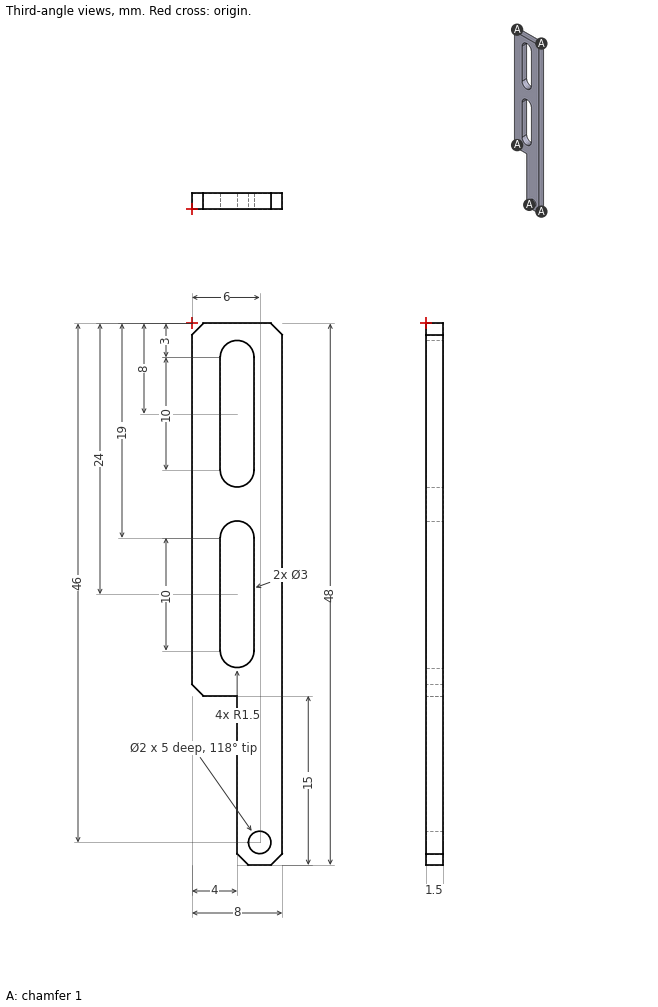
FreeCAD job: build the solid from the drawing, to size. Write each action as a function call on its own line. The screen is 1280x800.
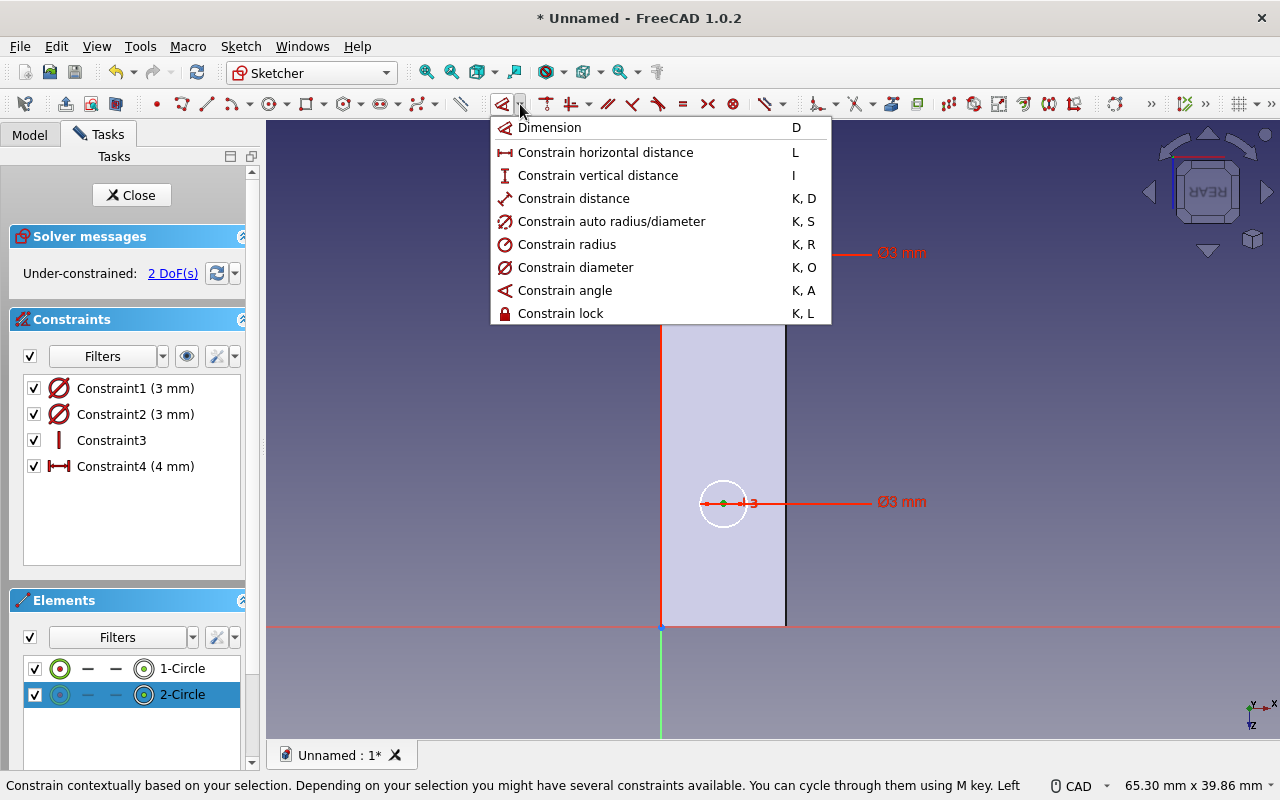
click(661, 176)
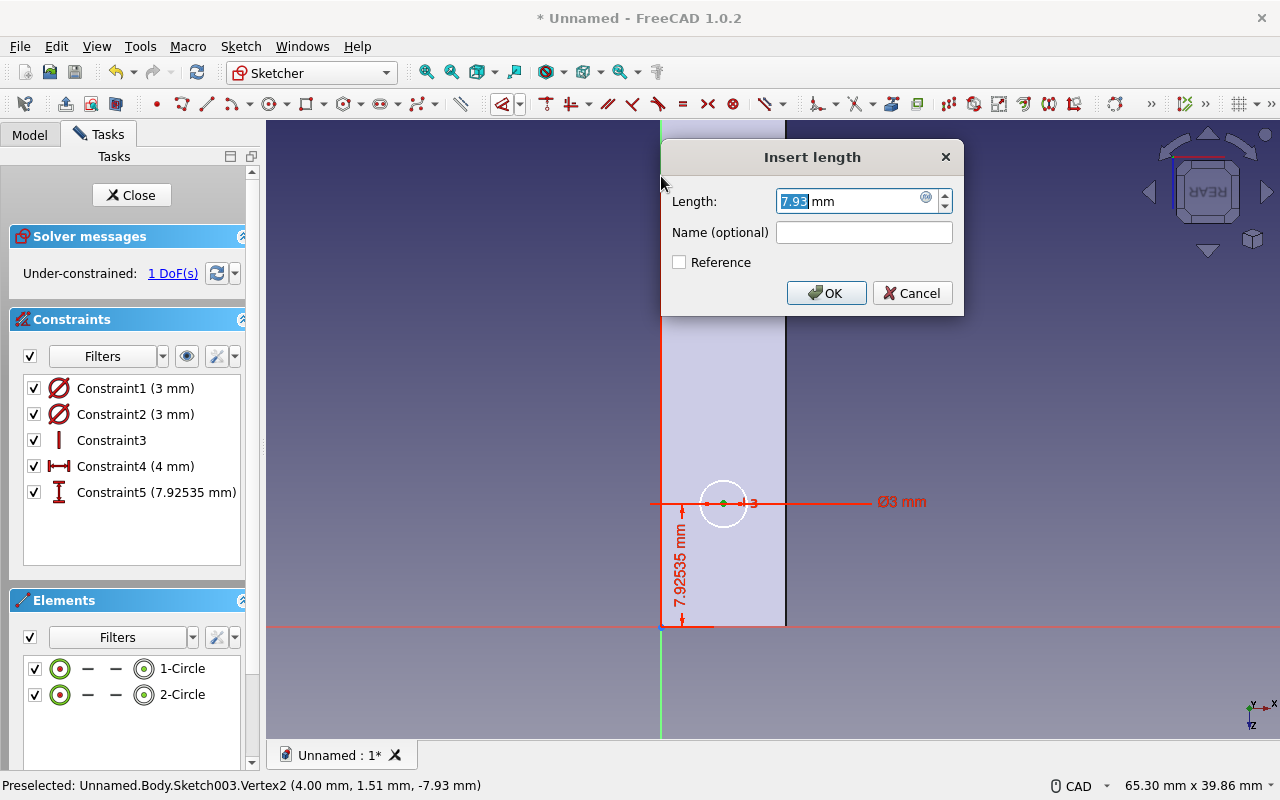
text(8)
key(Return)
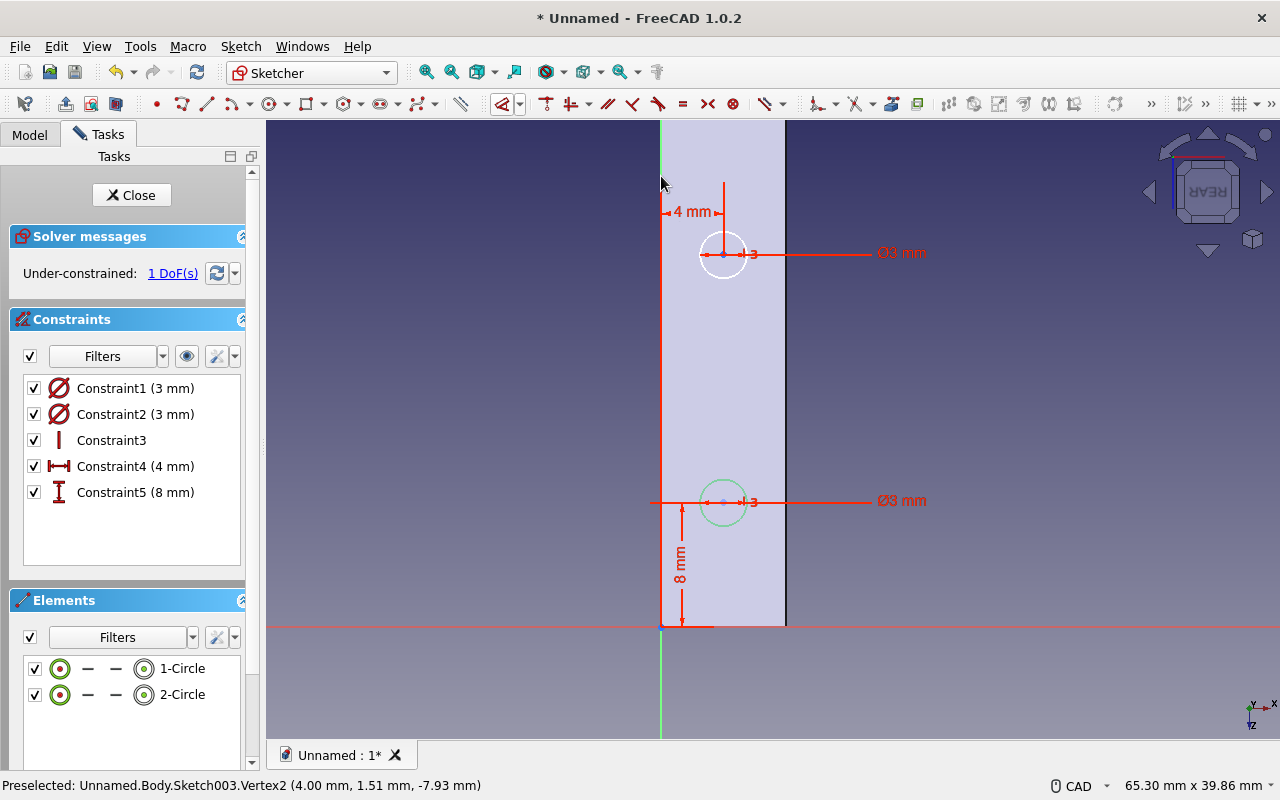
click(724, 255)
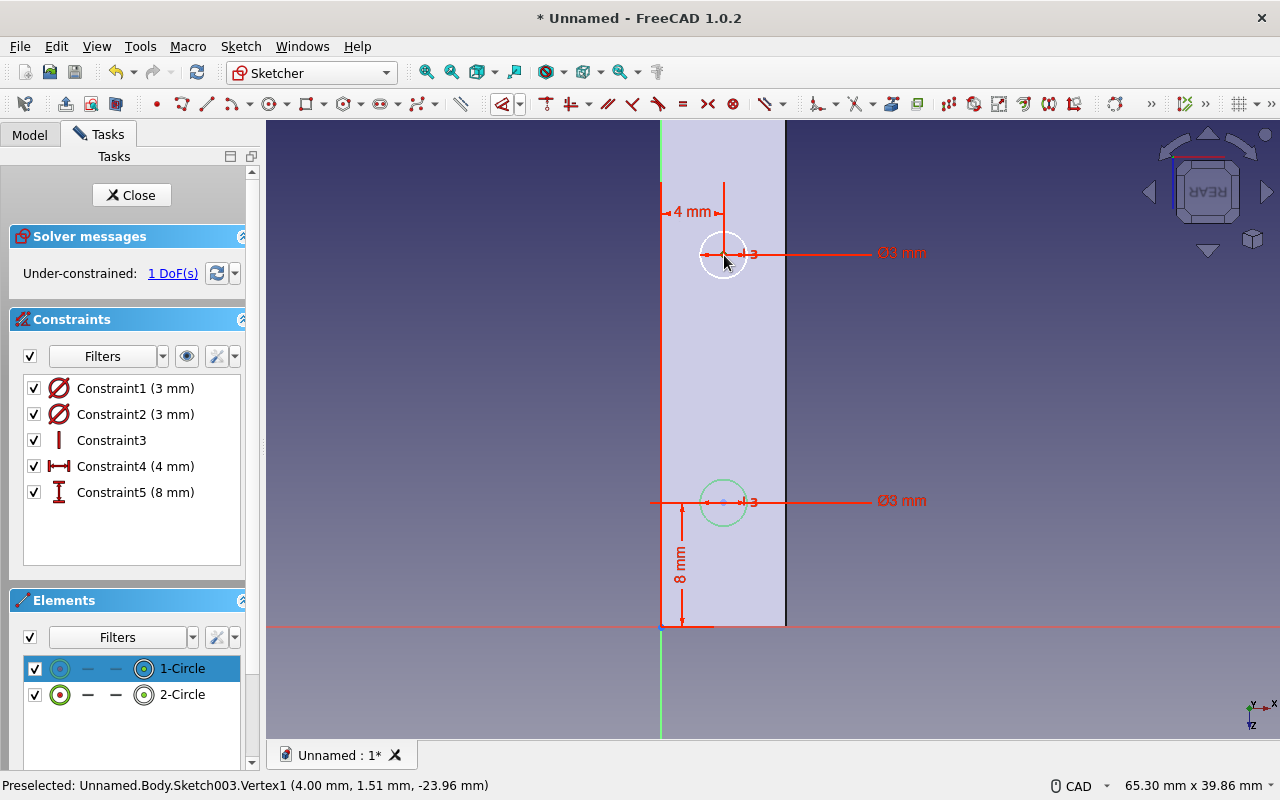
key(i)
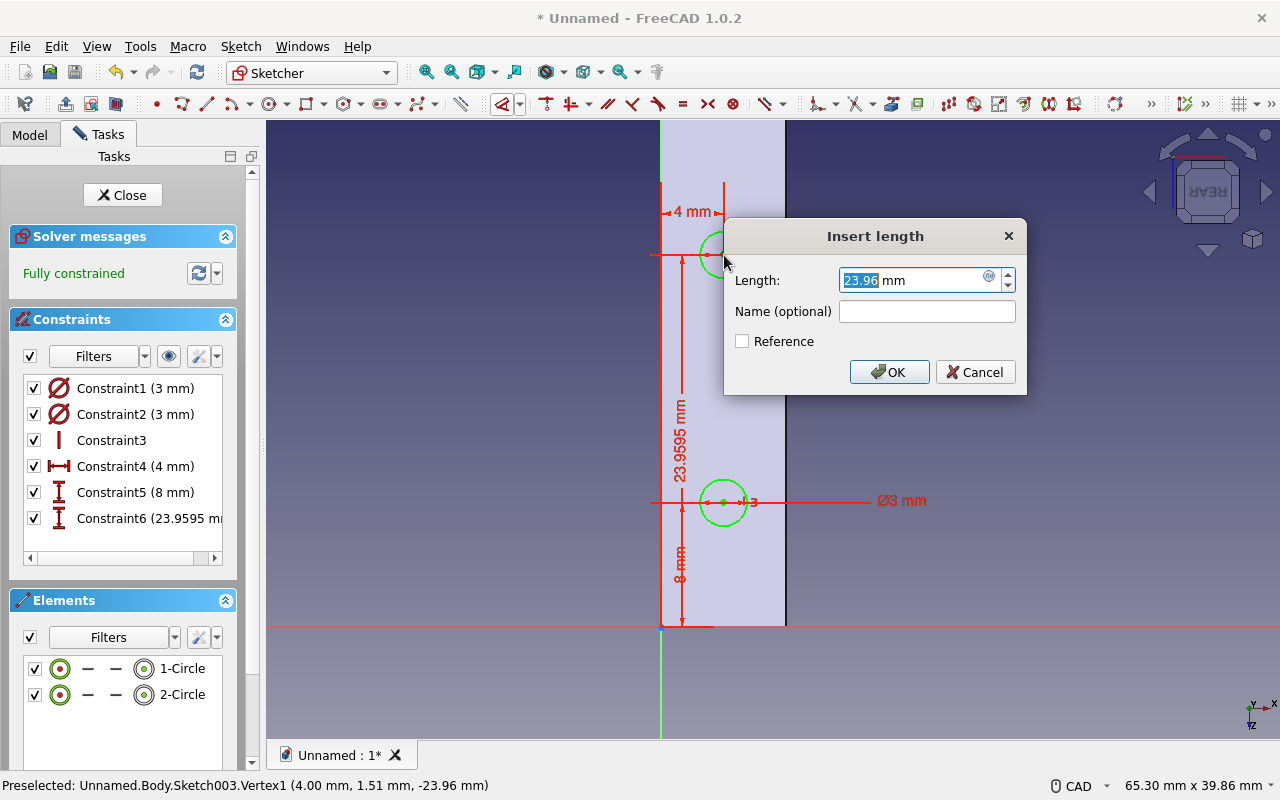
text(24)
key(Return)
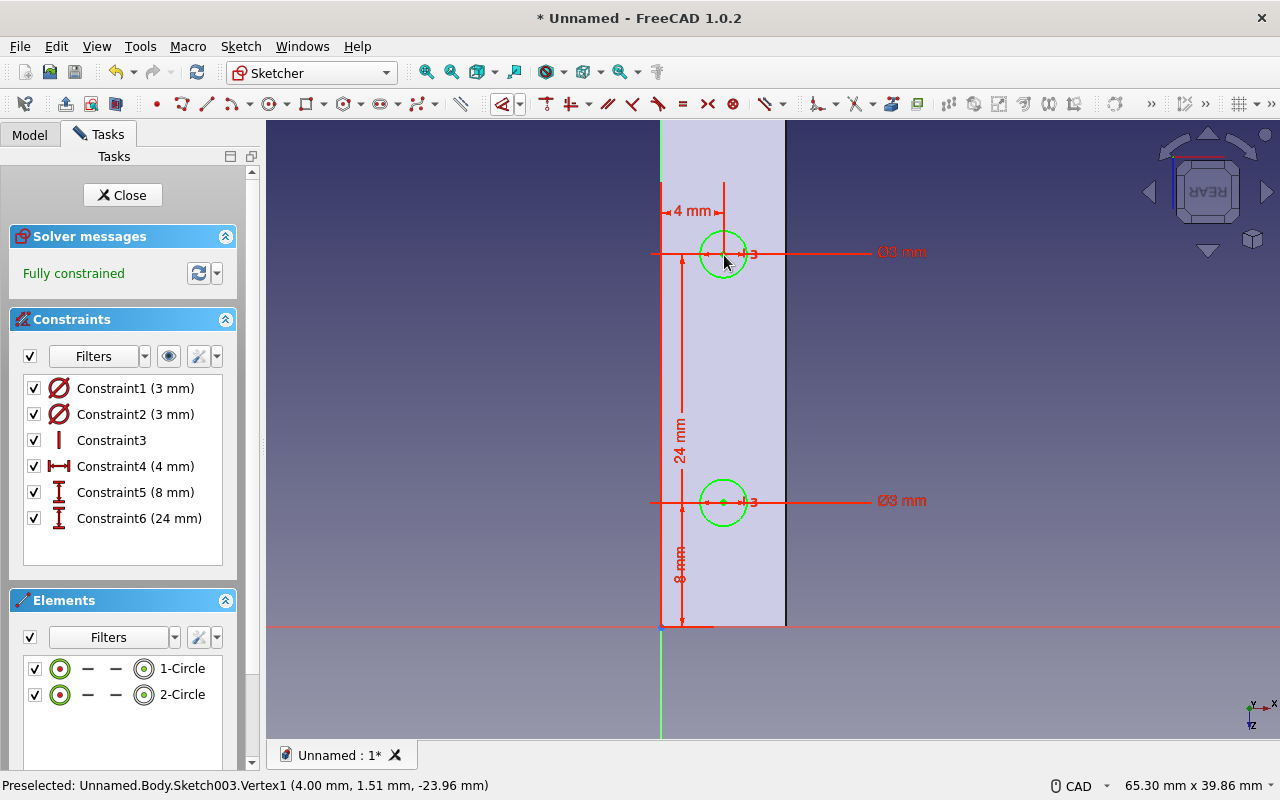
click(123, 195)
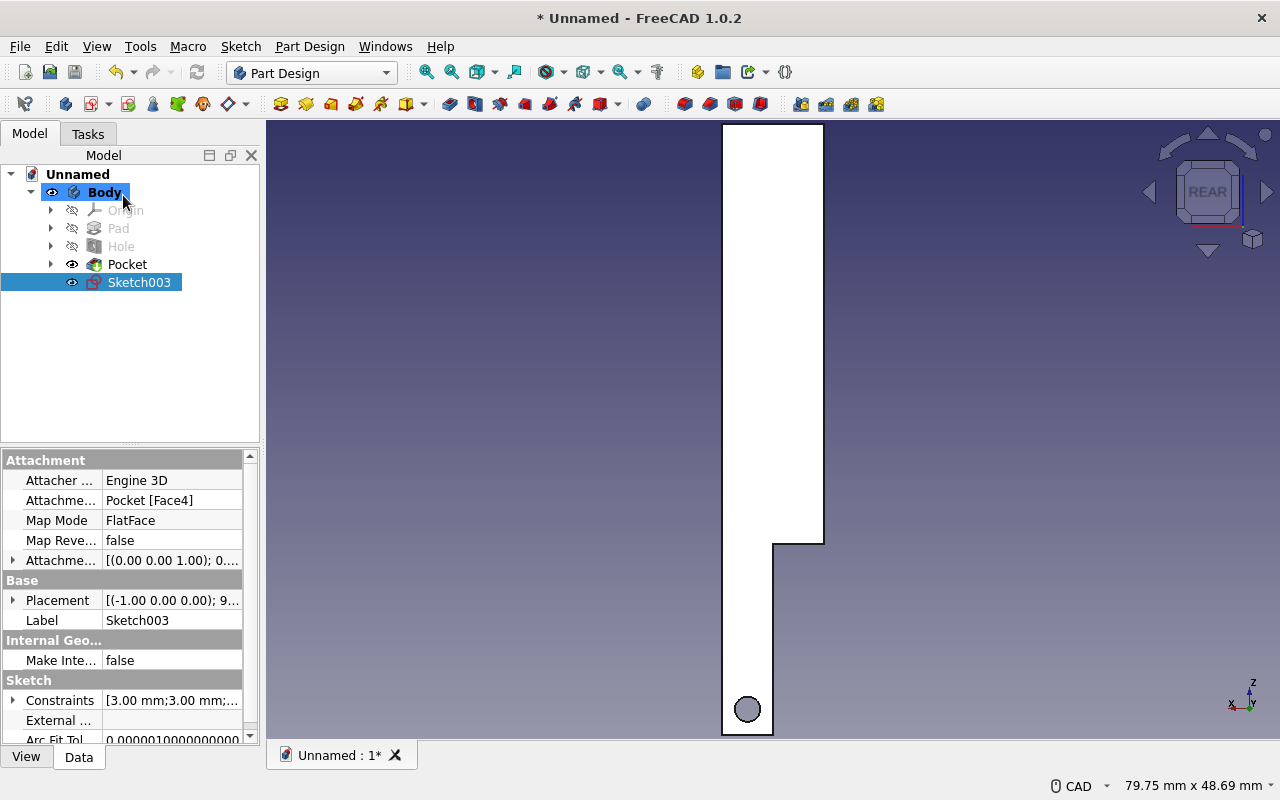
click(450, 104)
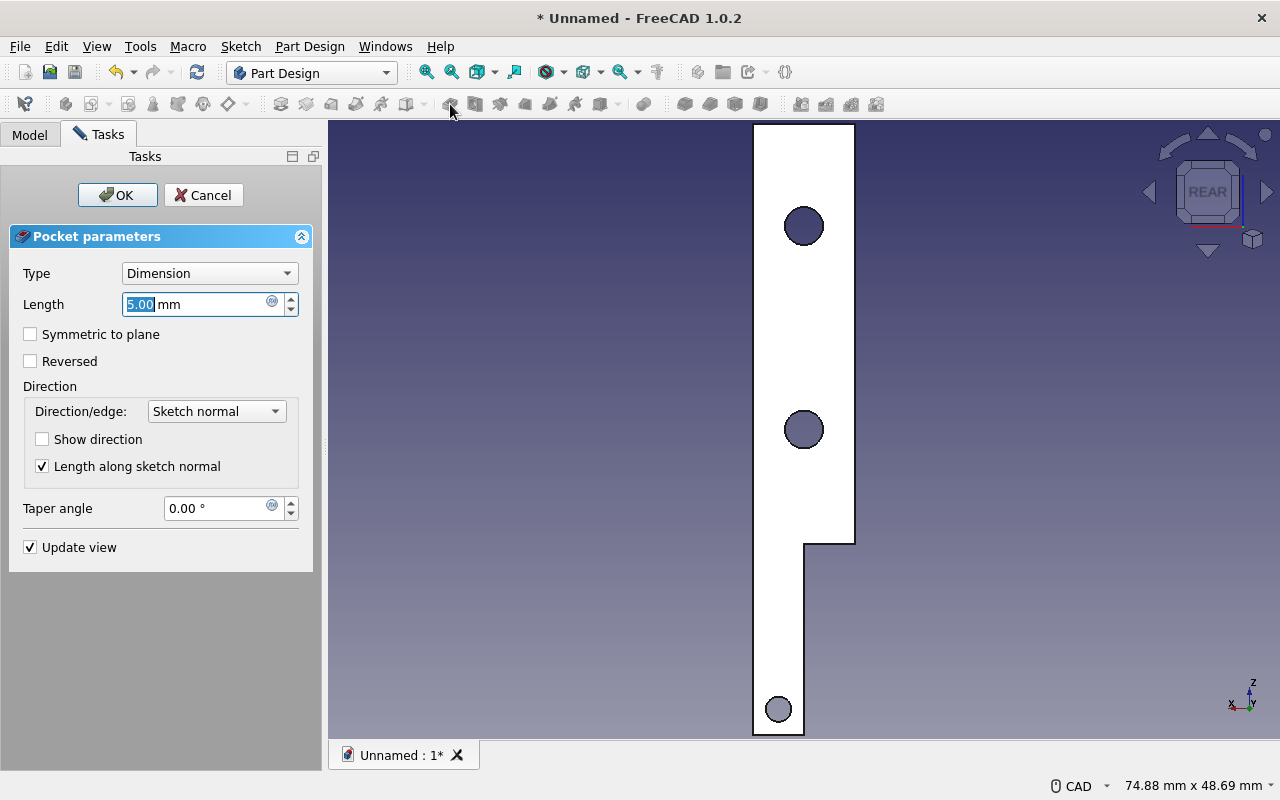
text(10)
key(Tab)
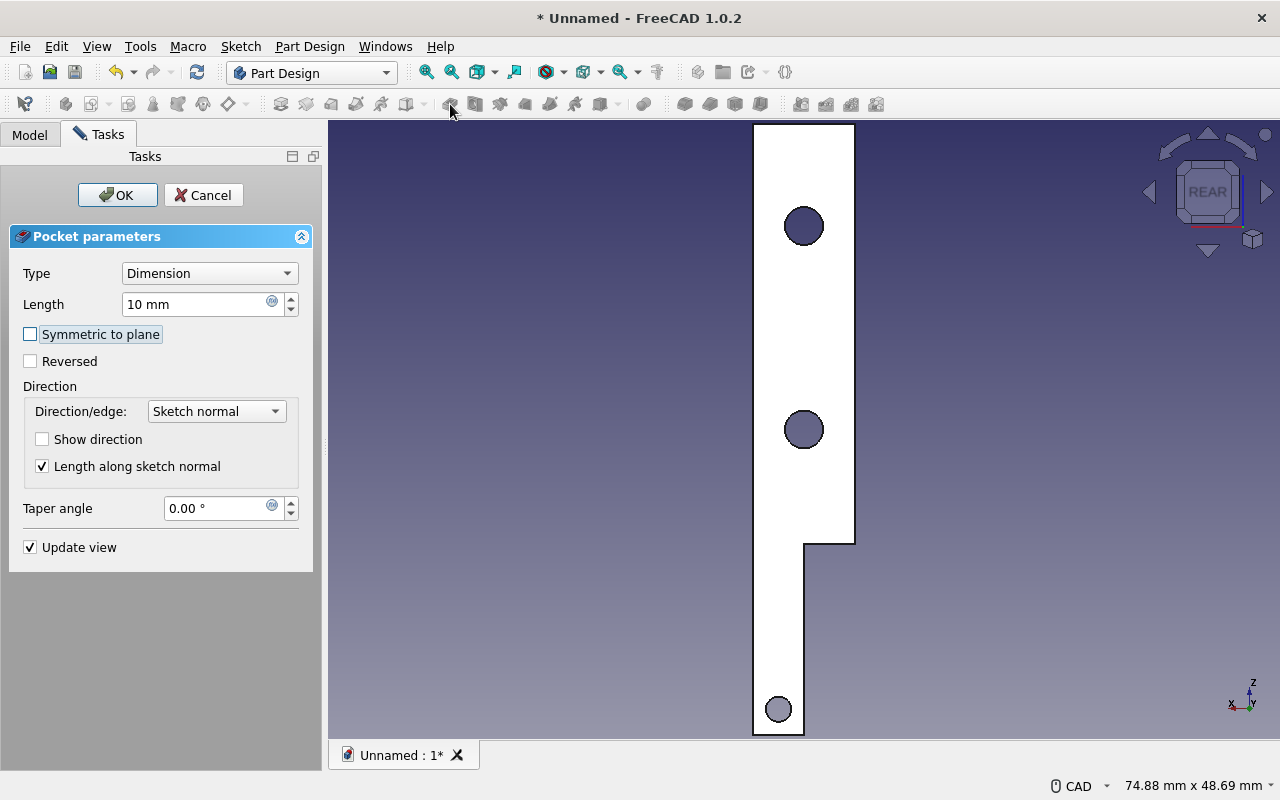
click(118, 195)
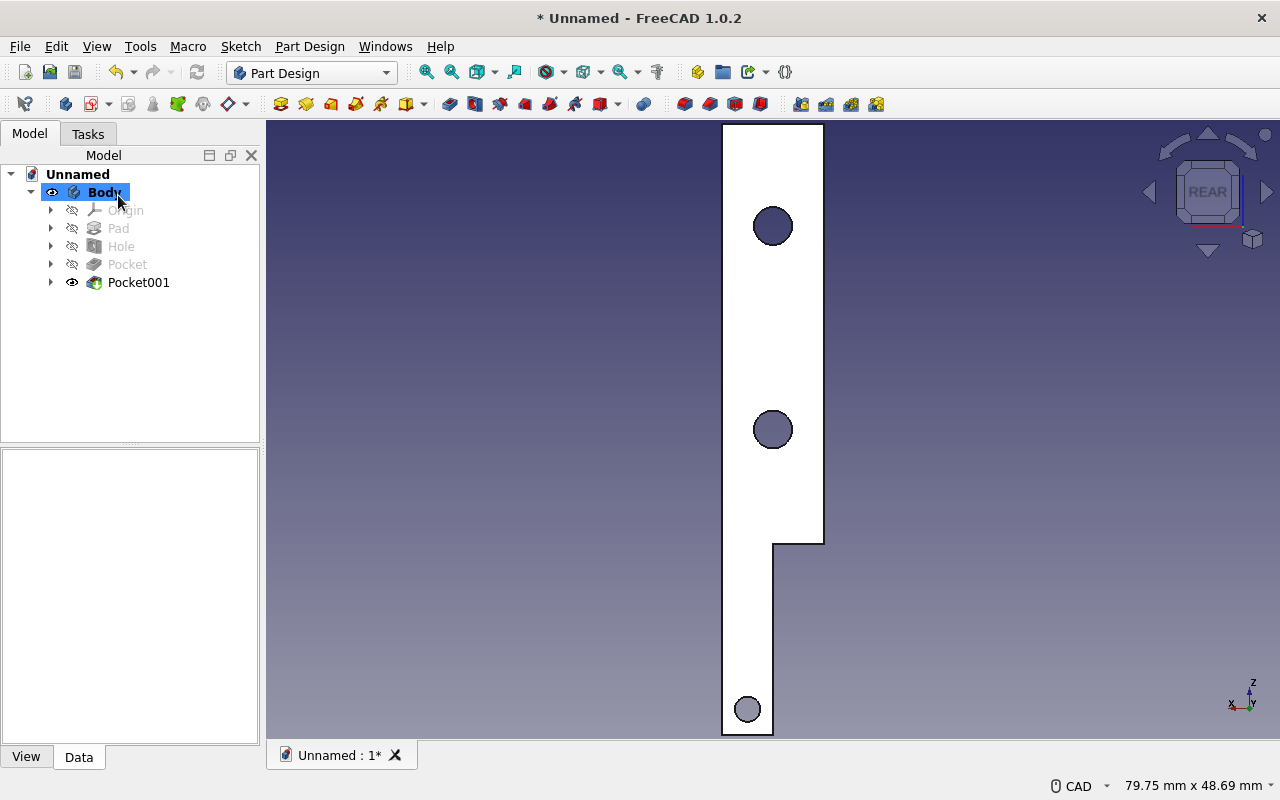
scroll(824, 543, up, 4)